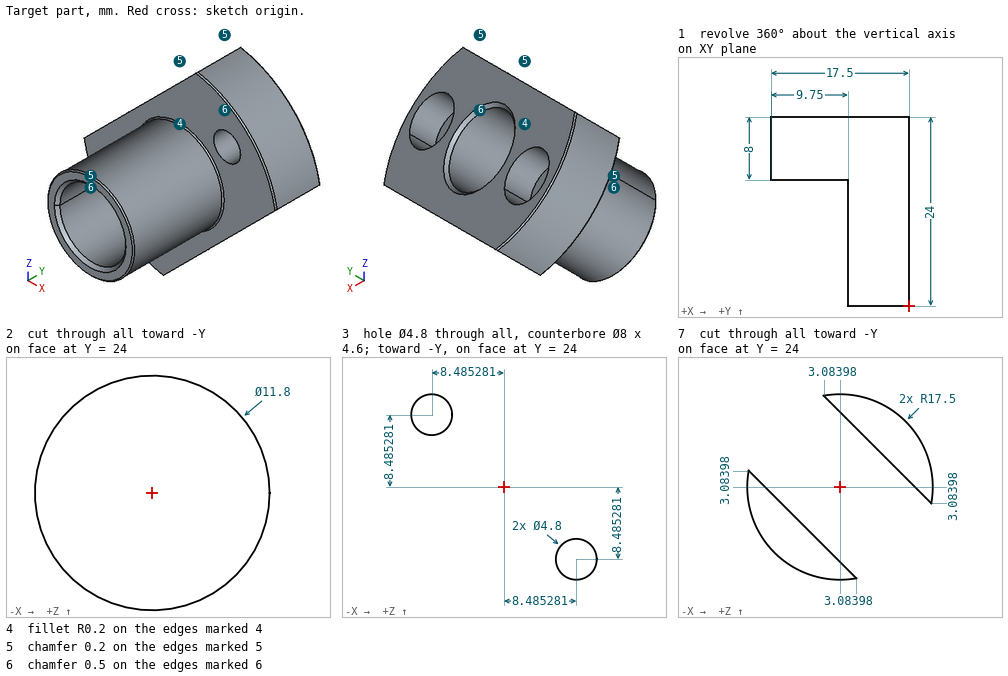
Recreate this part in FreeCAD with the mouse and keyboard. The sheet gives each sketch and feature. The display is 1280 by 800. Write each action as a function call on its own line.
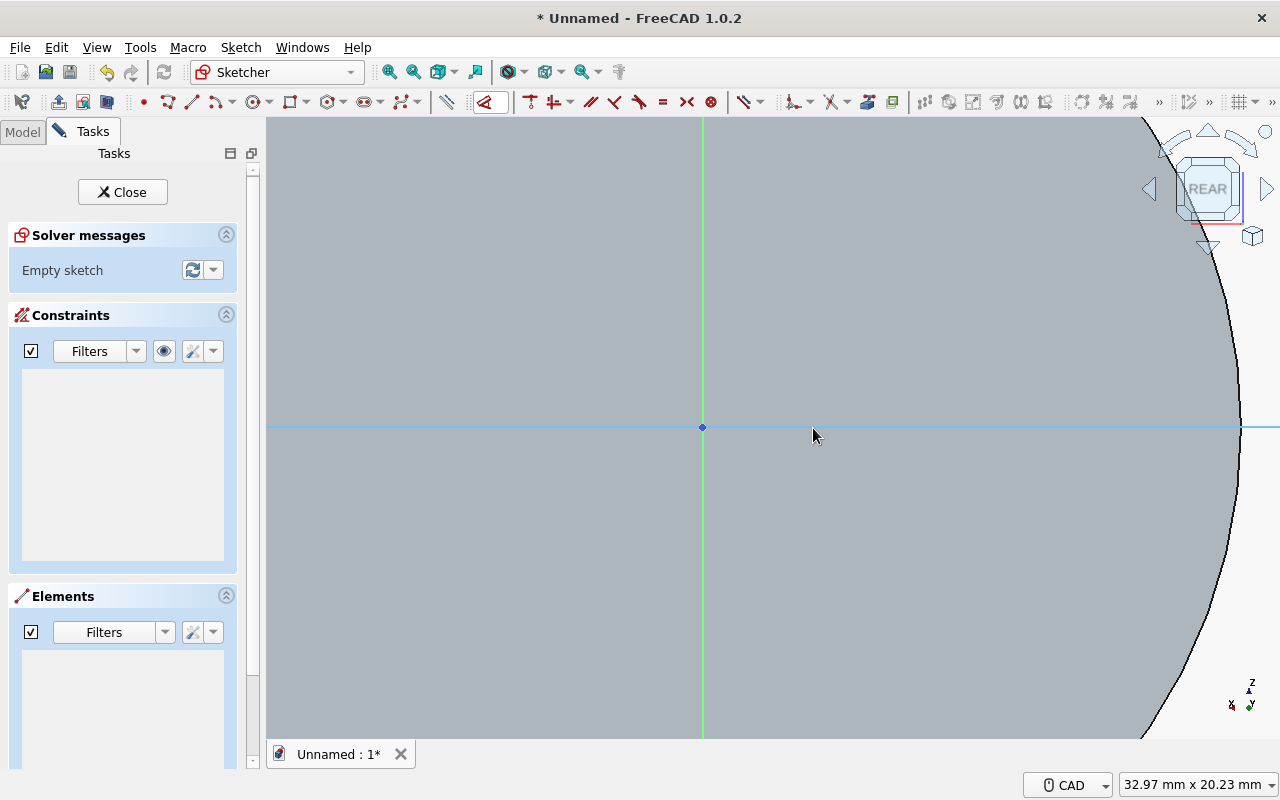
click(254, 102)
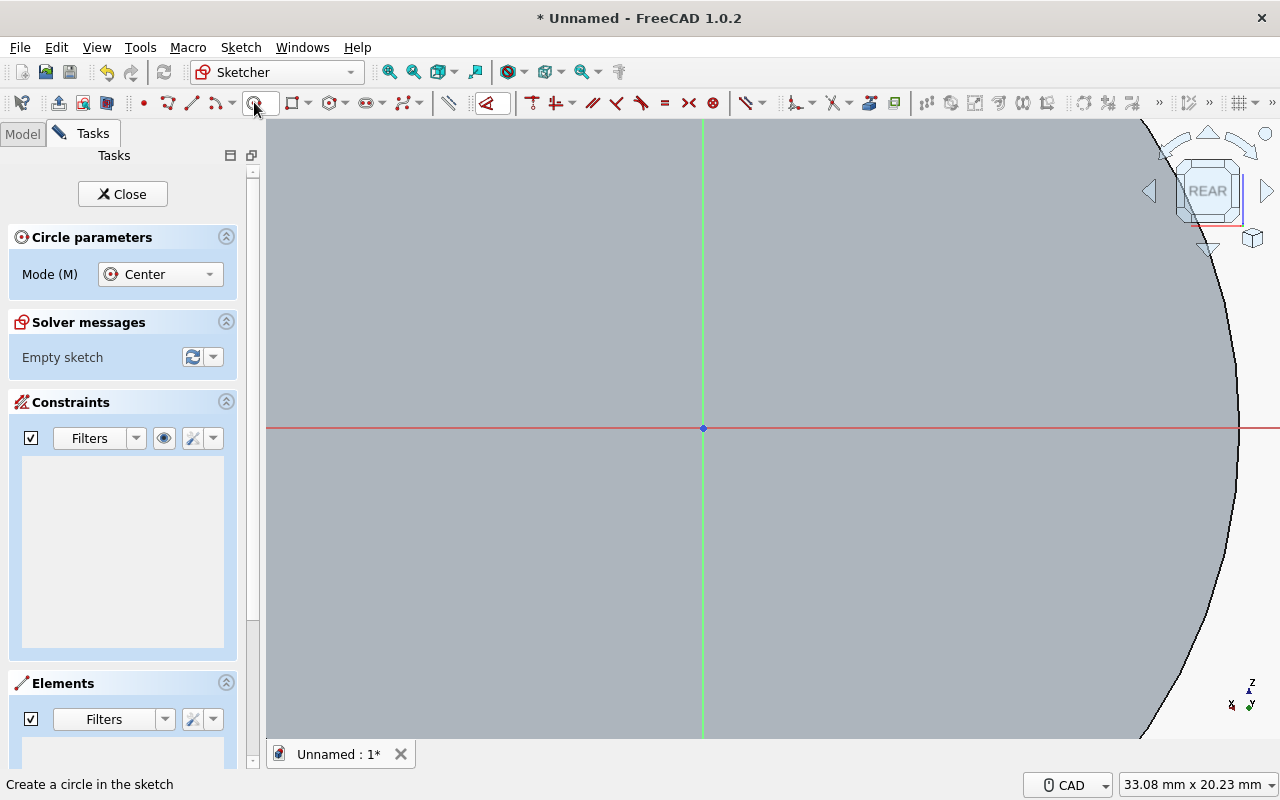
click(703, 428)
click(831, 300)
key(Escape)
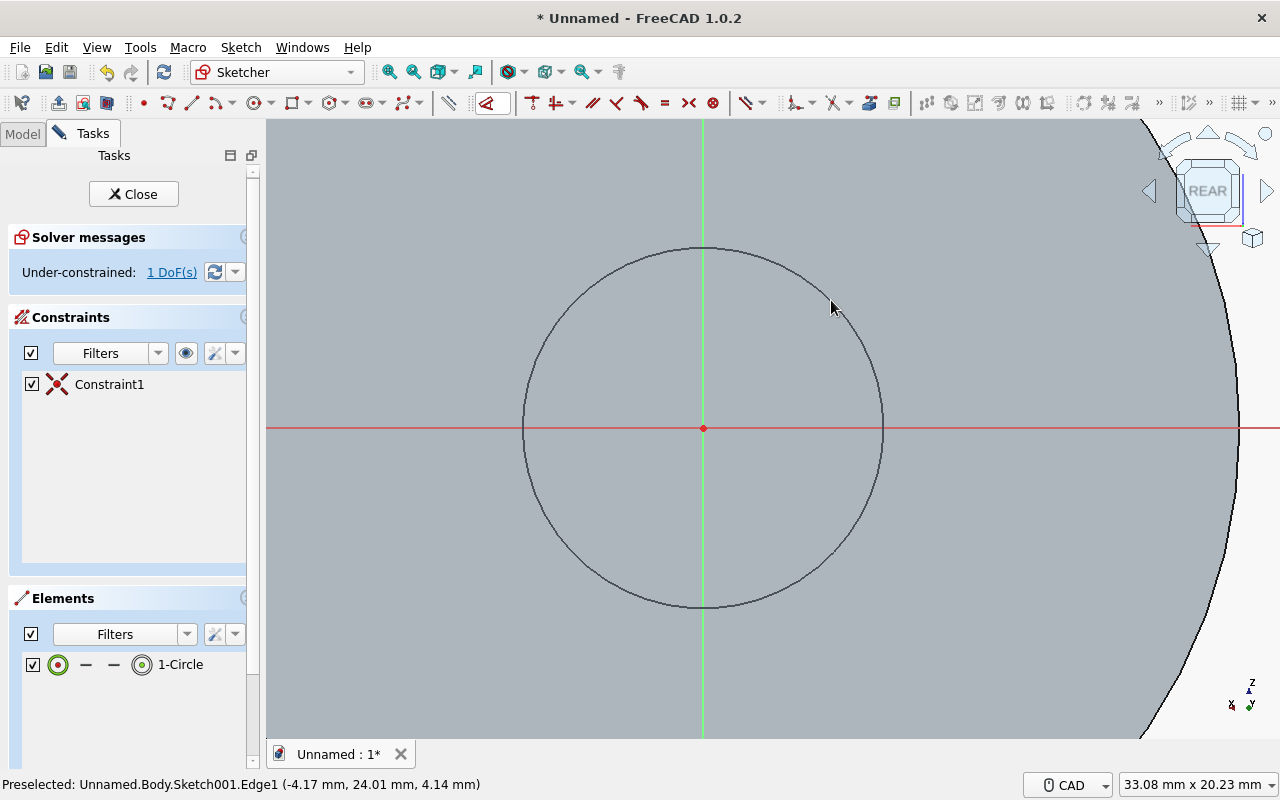
click(830, 300)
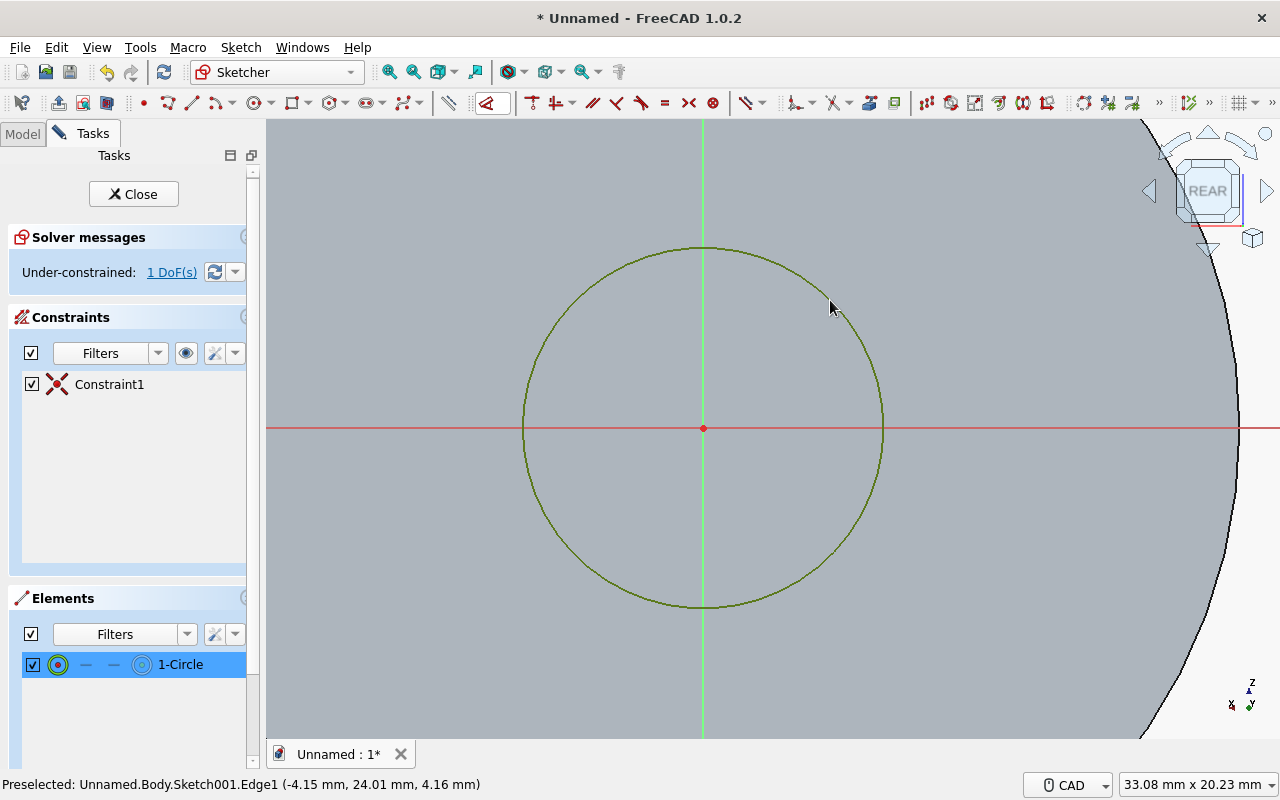
click(504, 104)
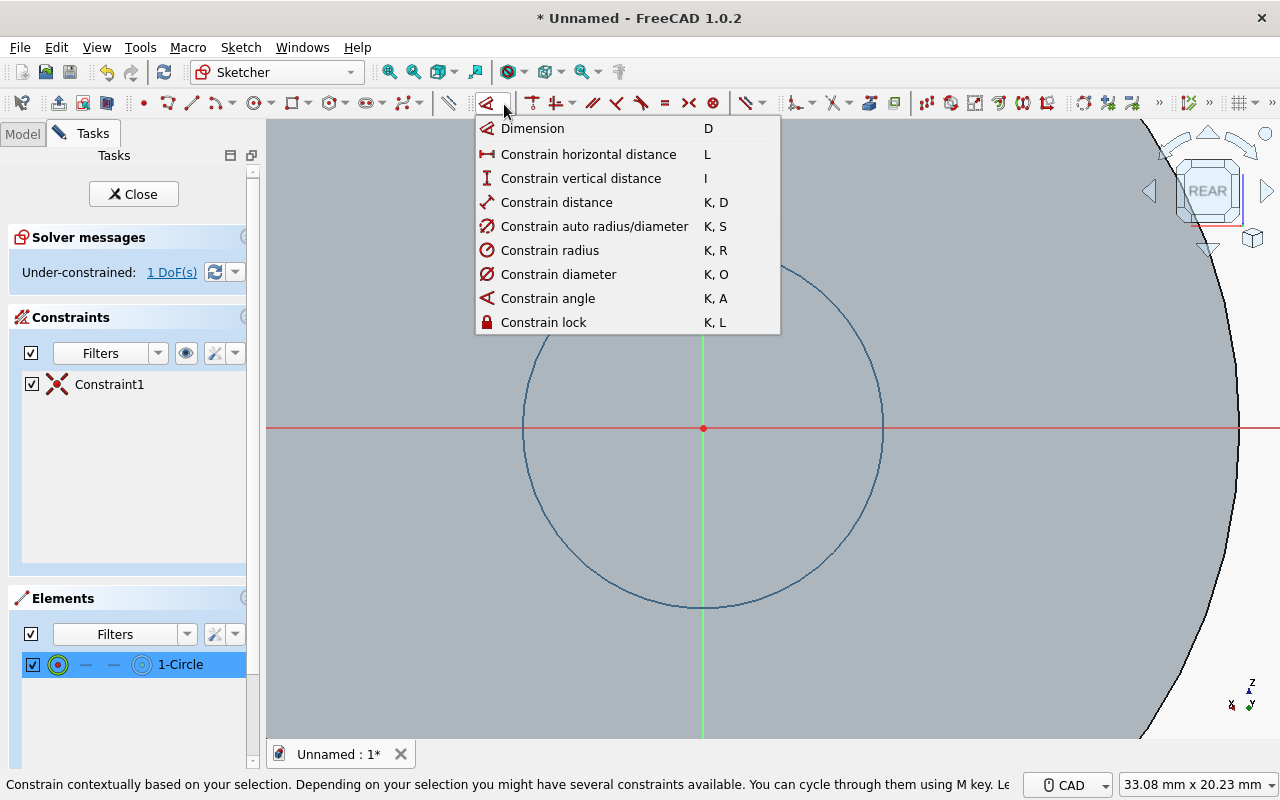
click(628, 274)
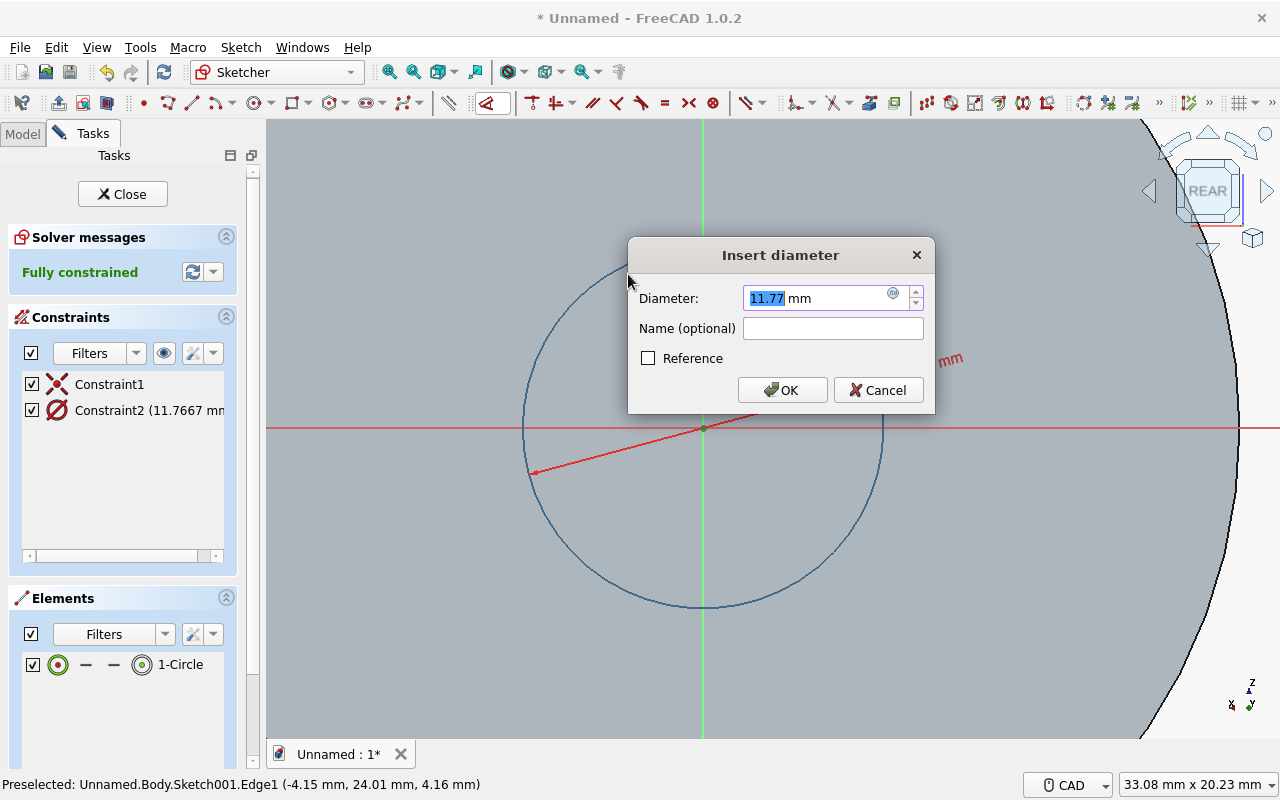
text(11.8)
key(Return)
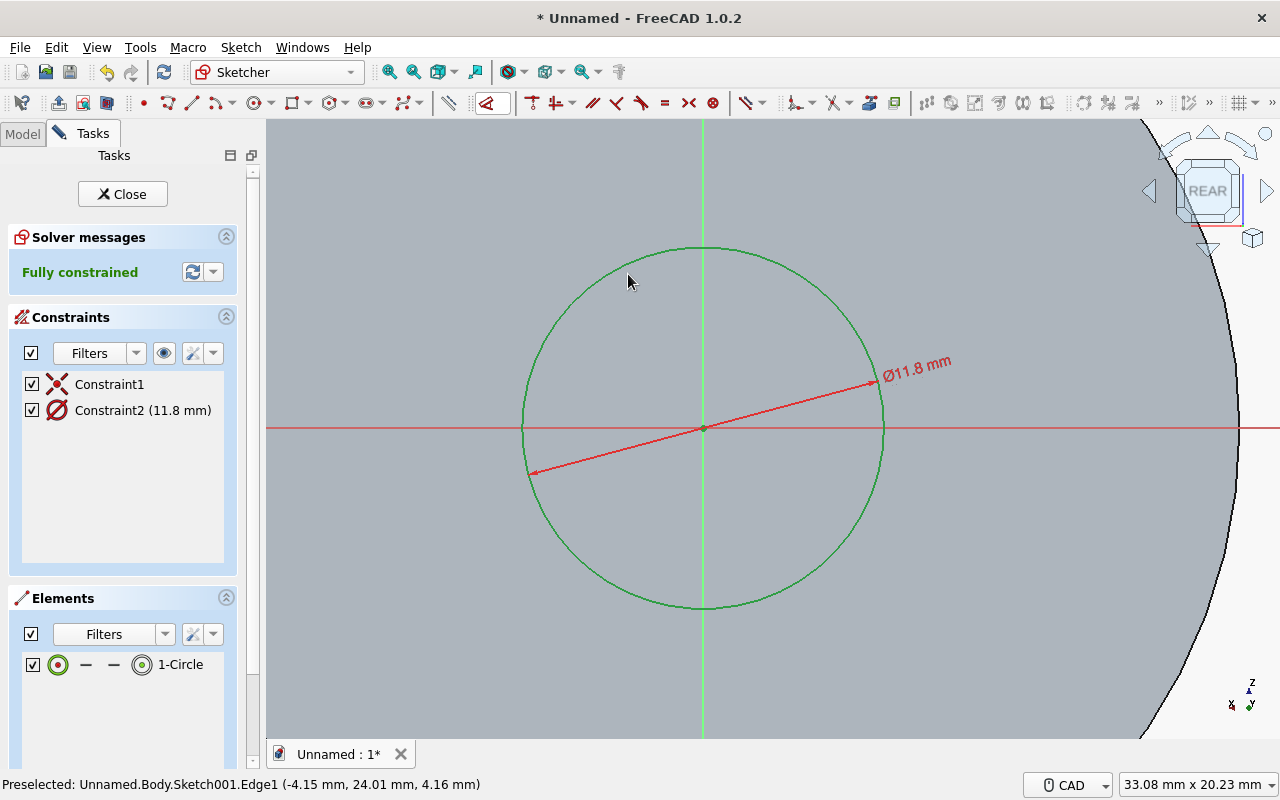
click(123, 194)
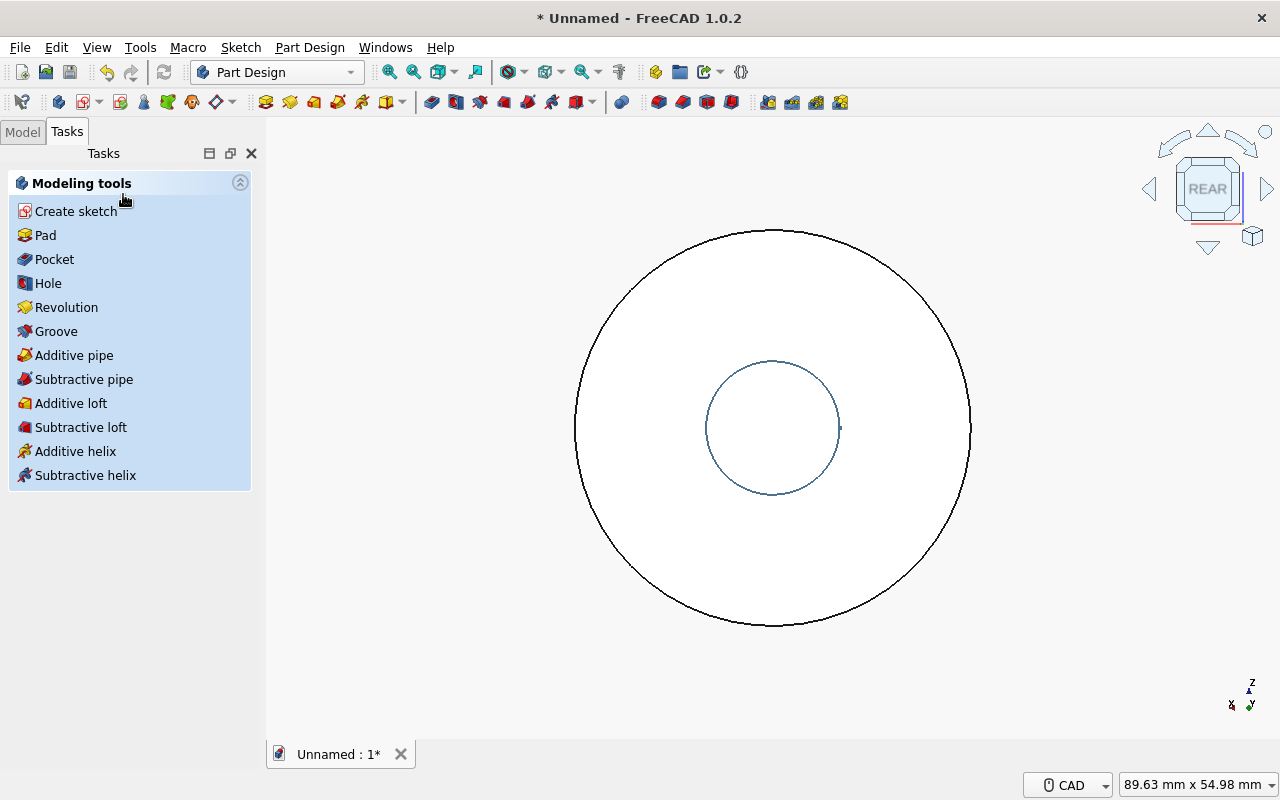
click(432, 102)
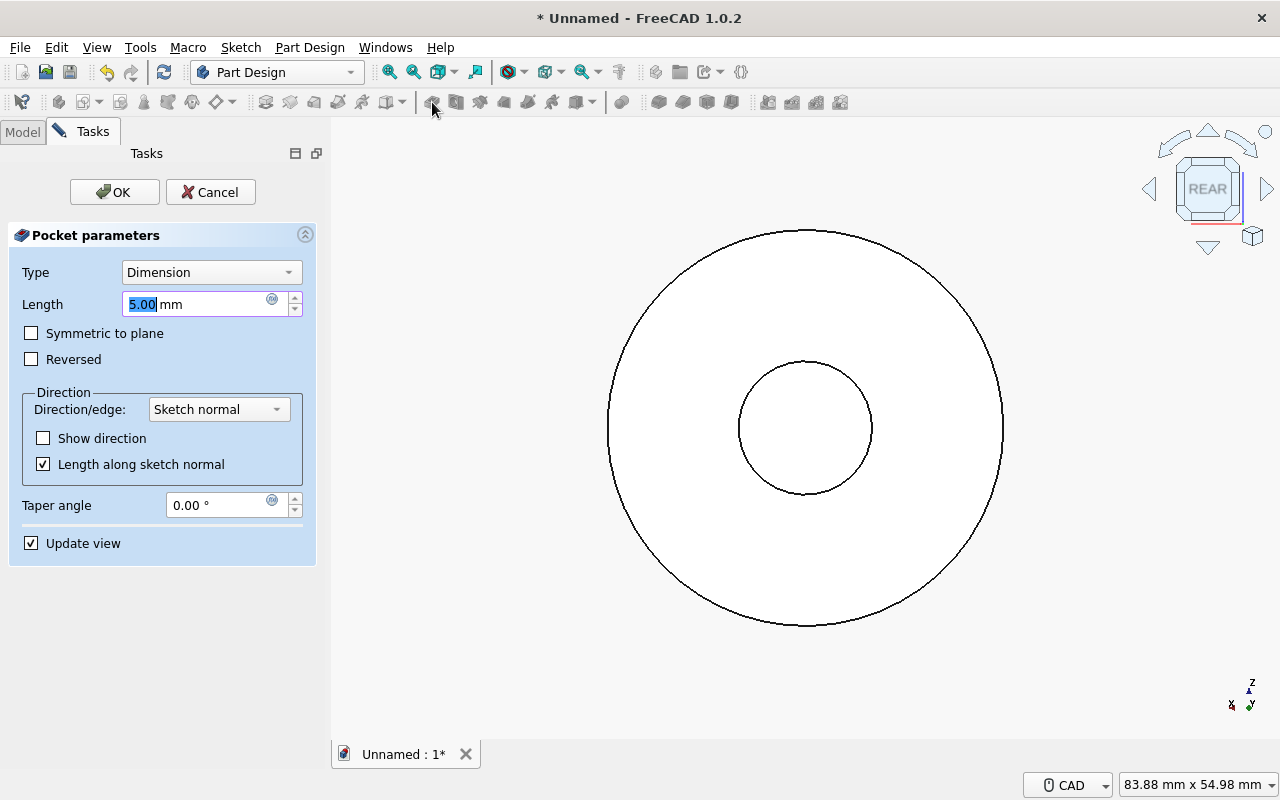
click(212, 272)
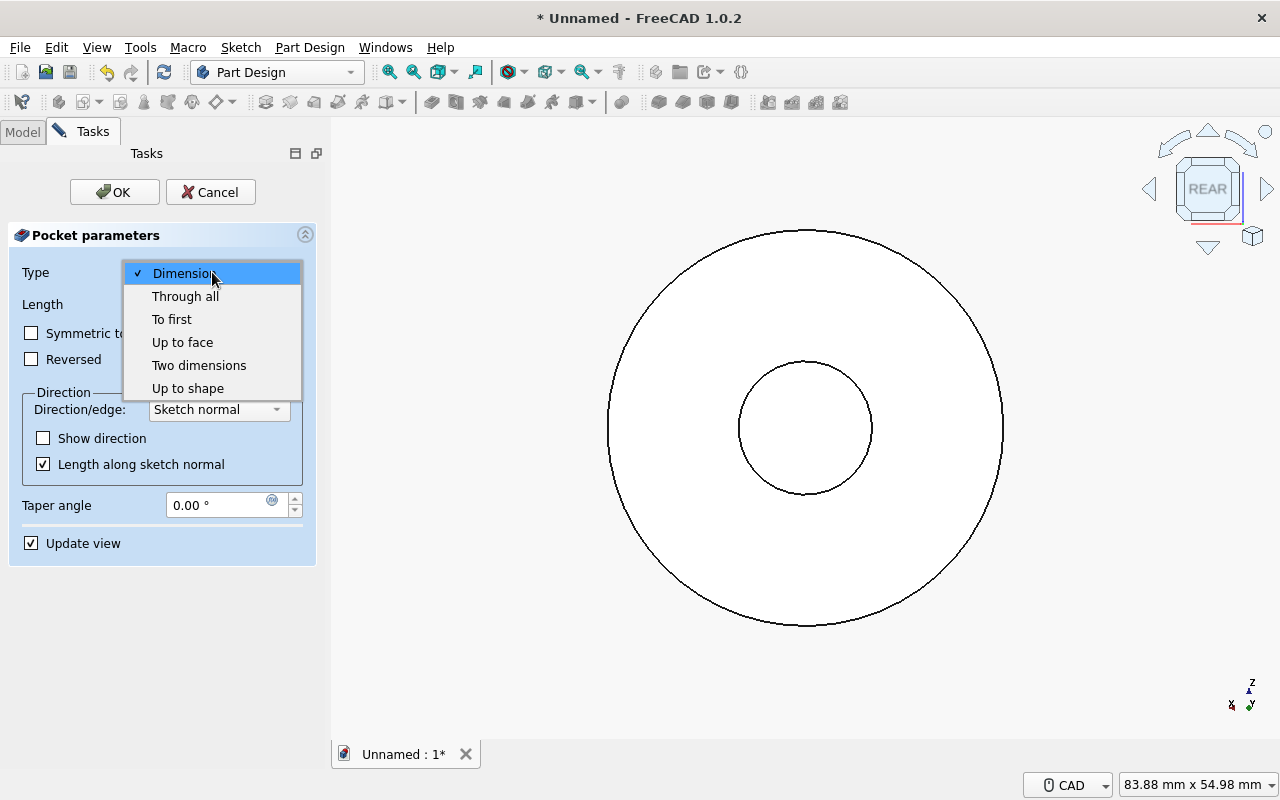
click(212, 296)